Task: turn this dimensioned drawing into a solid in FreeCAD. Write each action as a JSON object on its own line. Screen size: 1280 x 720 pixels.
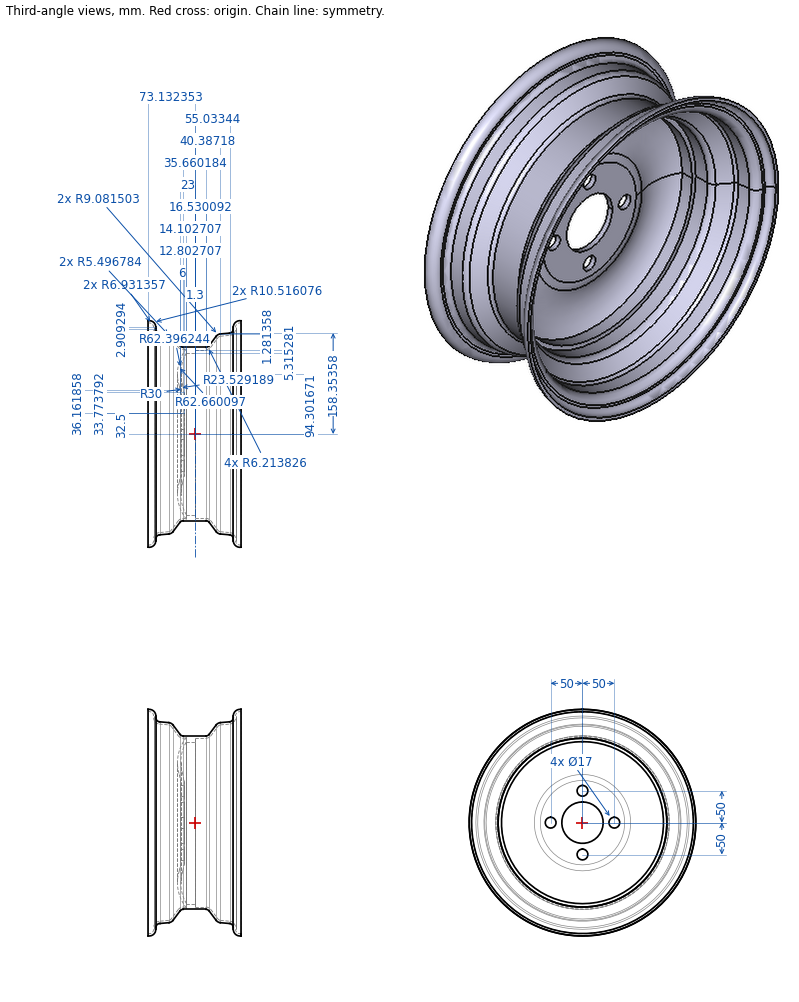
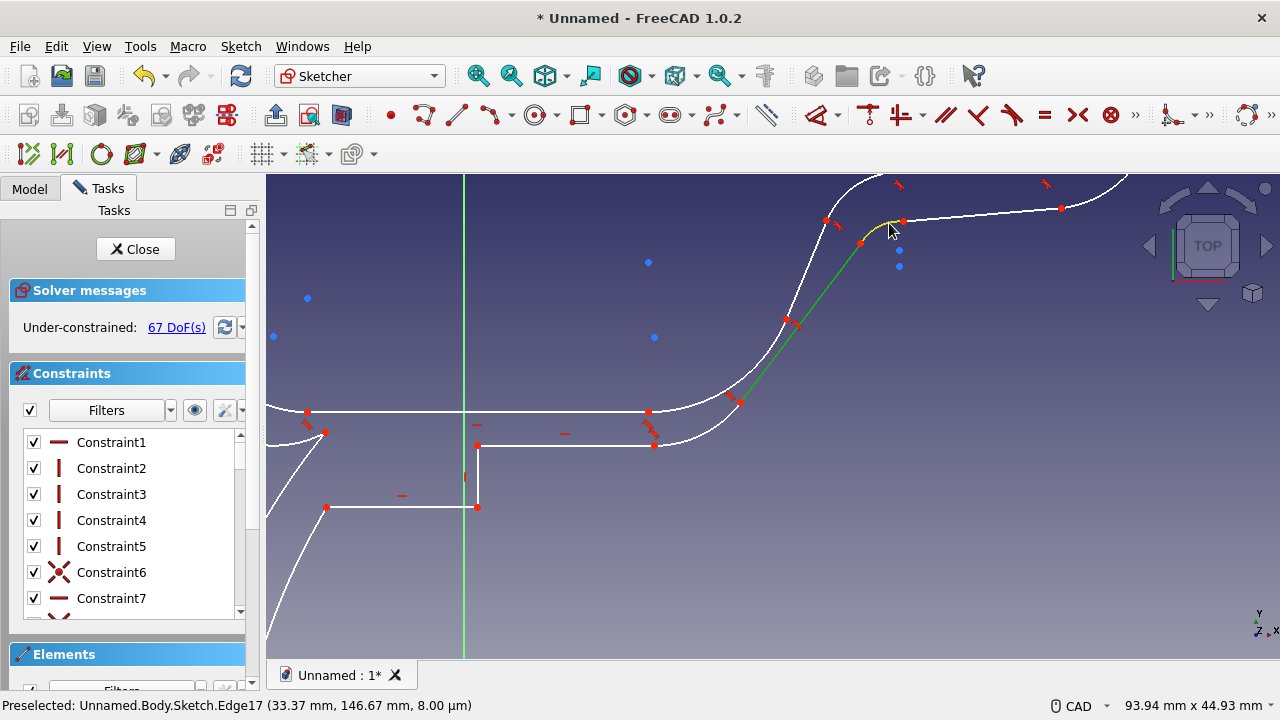
{"action": "left_click", "coordinate": [888, 223]}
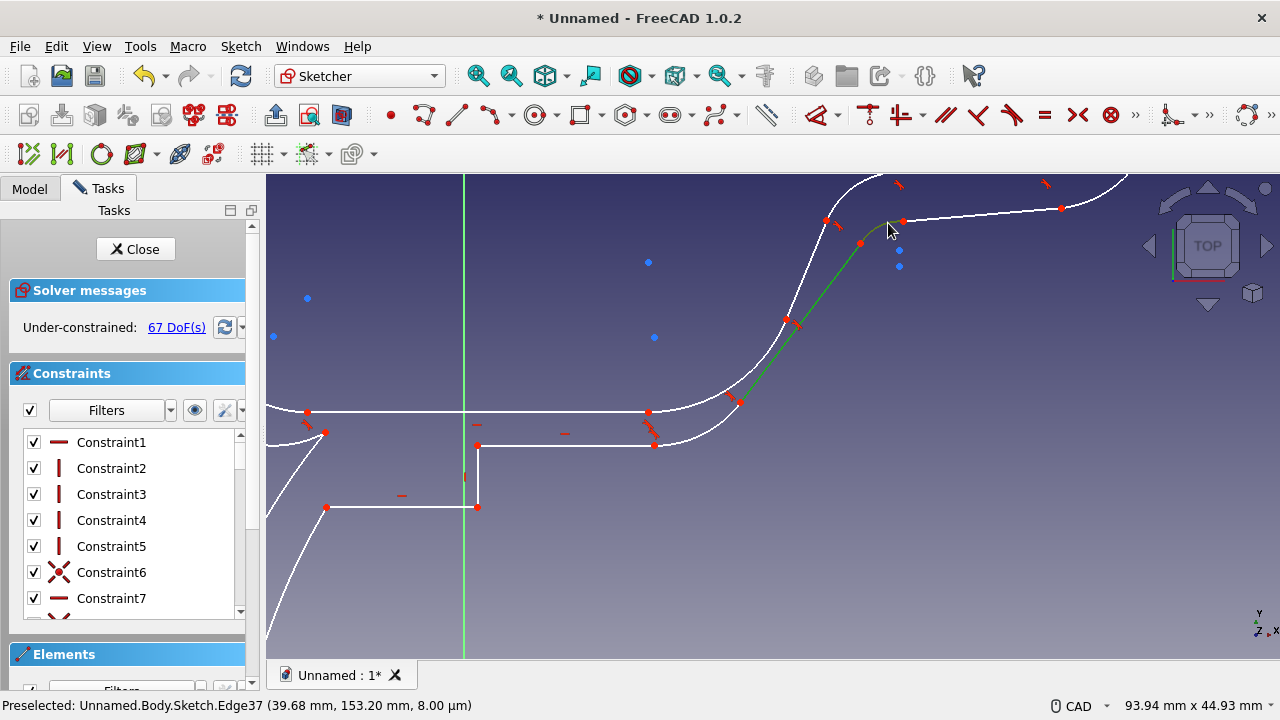
{"action": "key", "text": "t"}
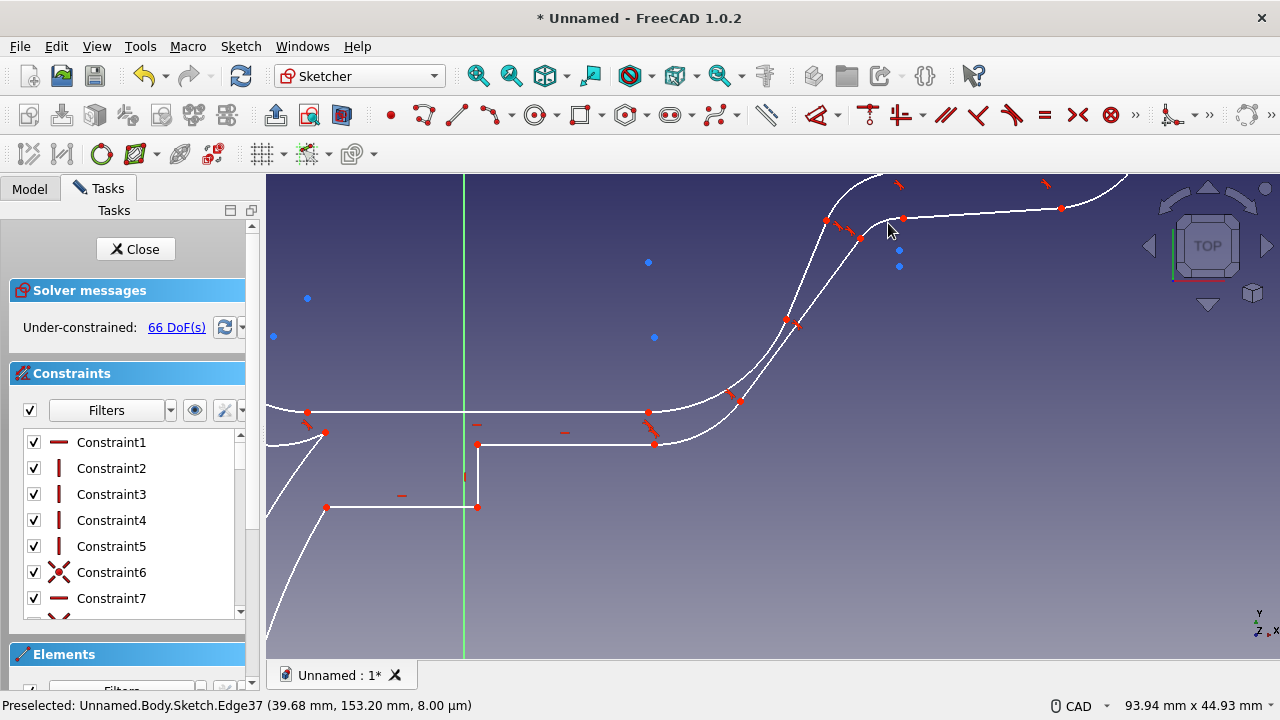
{"action": "scroll", "coordinate": [752, 318], "scroll_direction": "down", "scroll_amount": 9}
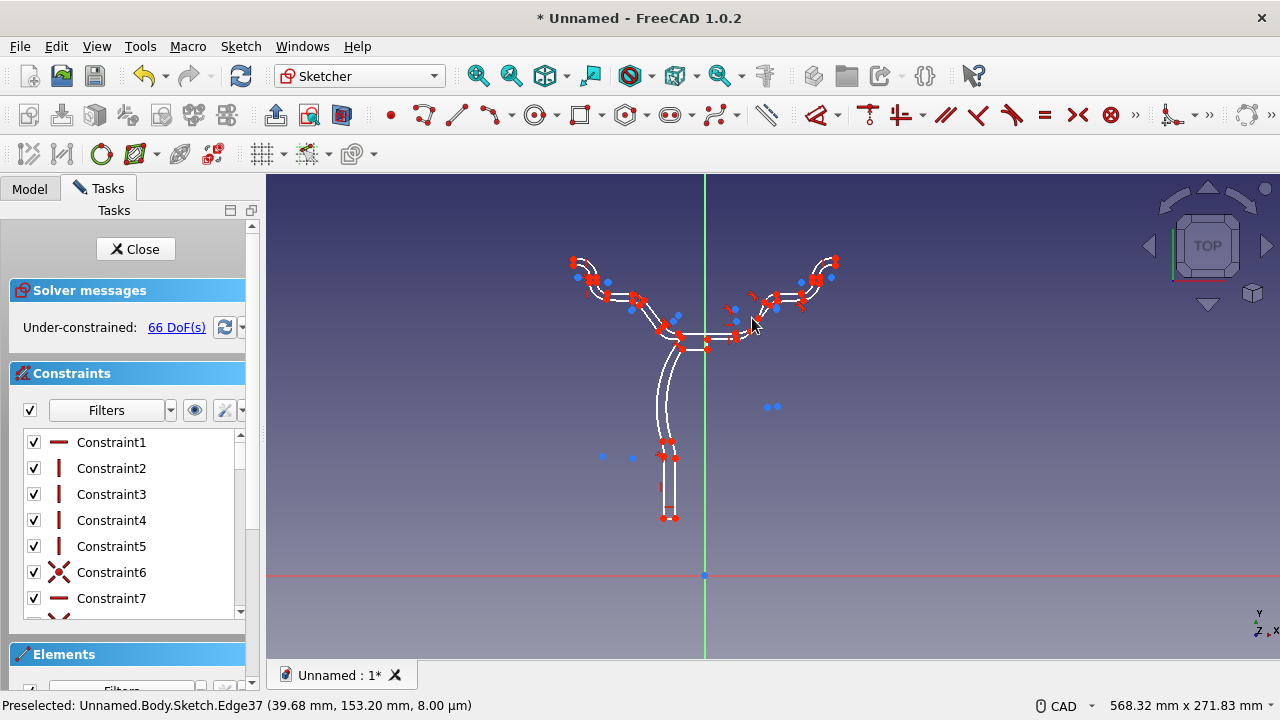
{"action": "scroll", "coordinate": [785, 301], "scroll_direction": "up", "scroll_amount": 4}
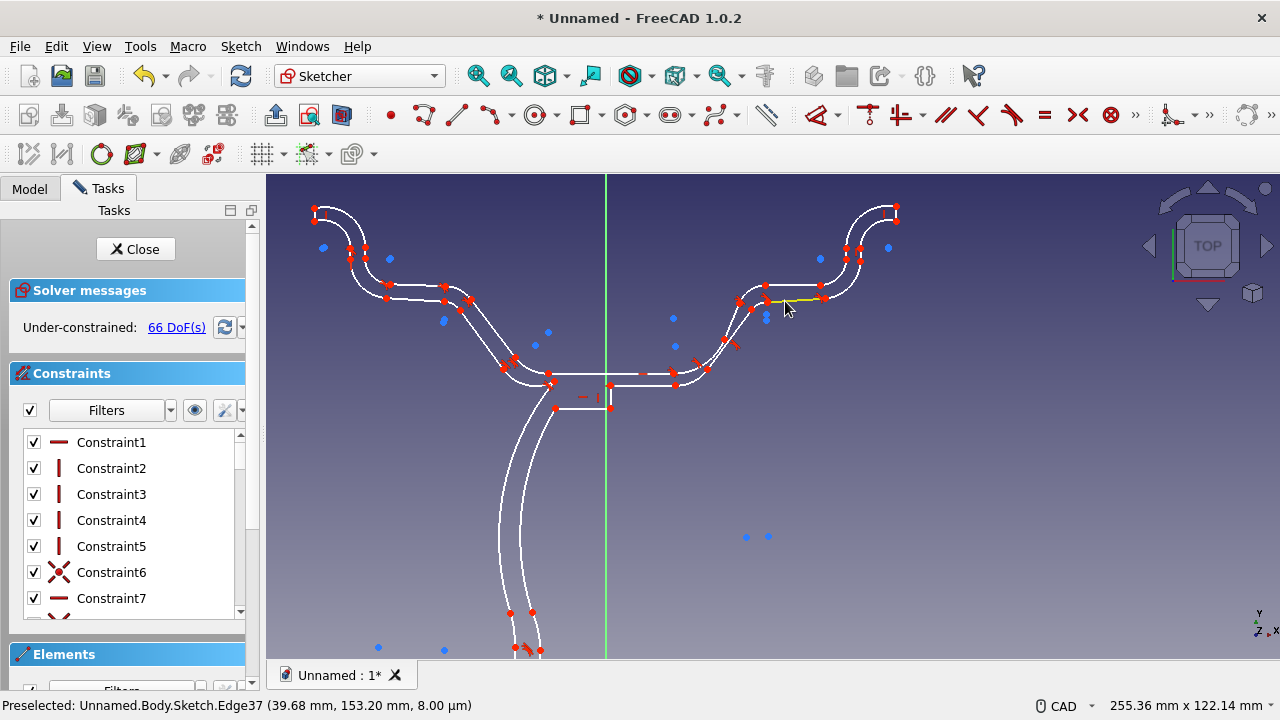
{"action": "left_click", "coordinate": [785, 301]}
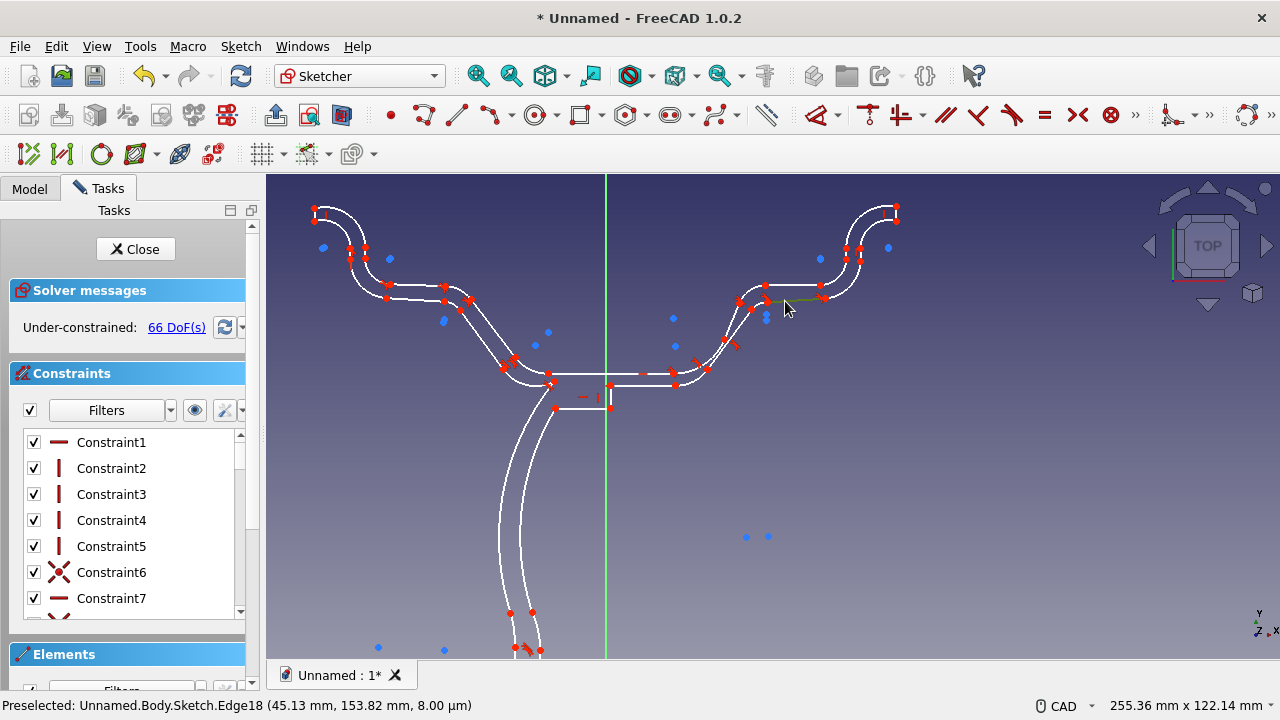
{"action": "scroll", "coordinate": [759, 304], "scroll_direction": "up", "scroll_amount": 3}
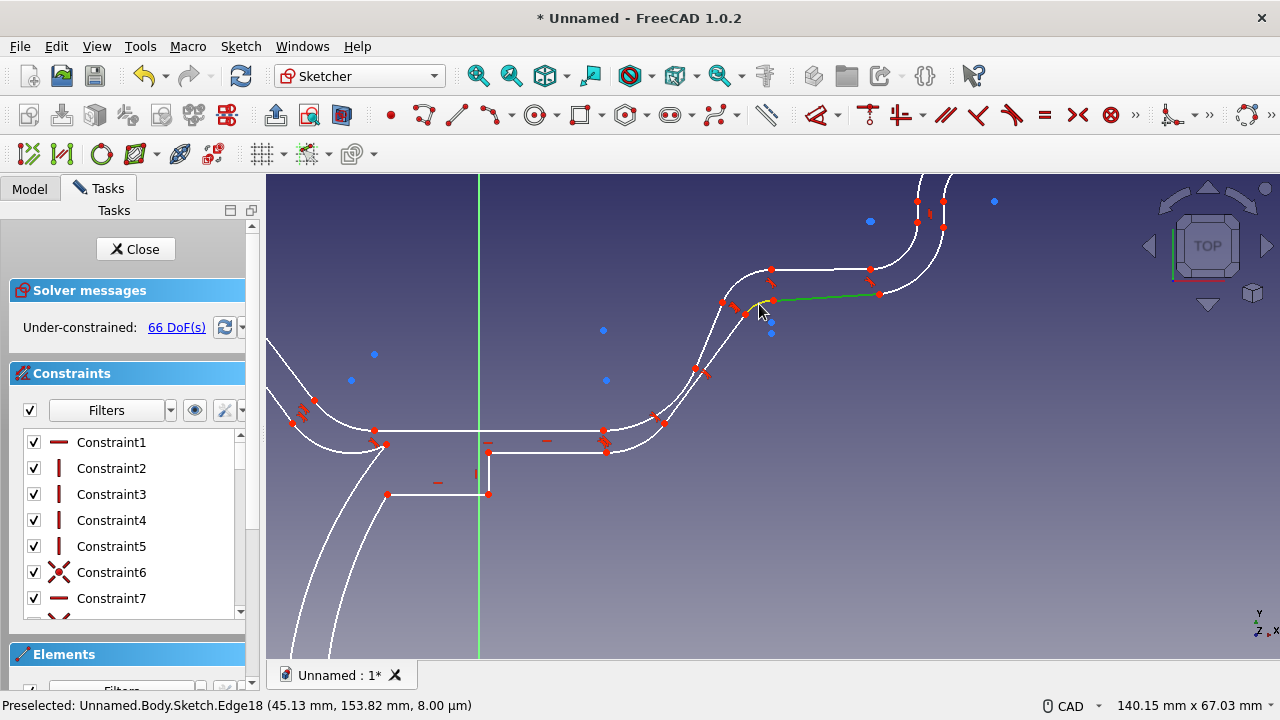
{"action": "left_click", "coordinate": [758, 304]}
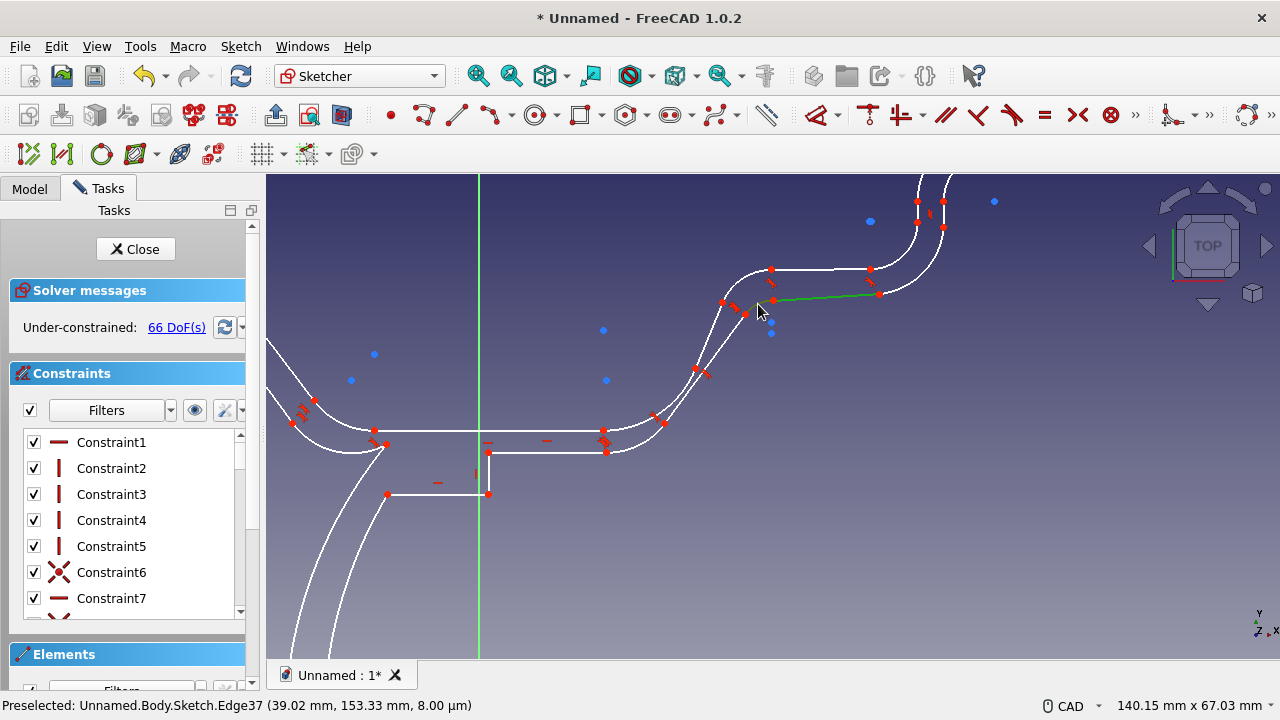
{"action": "key", "text": "t"}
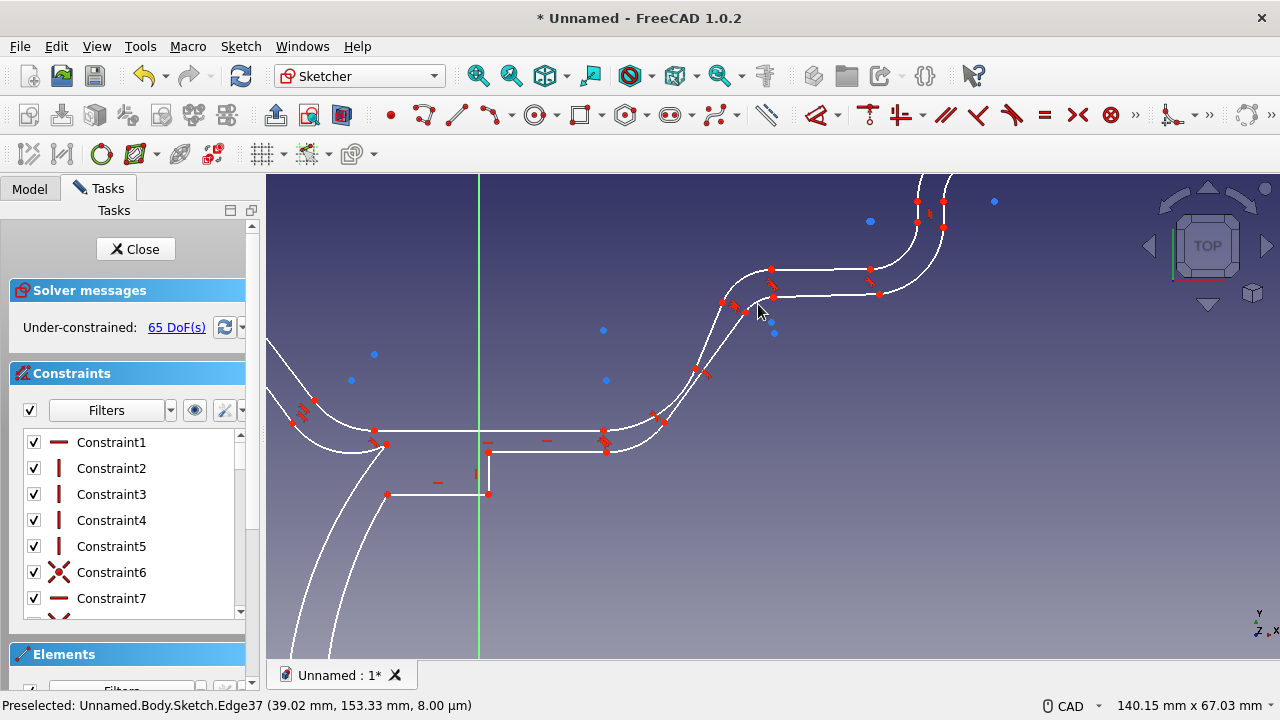
{"action": "left_click", "coordinate": [806, 296]}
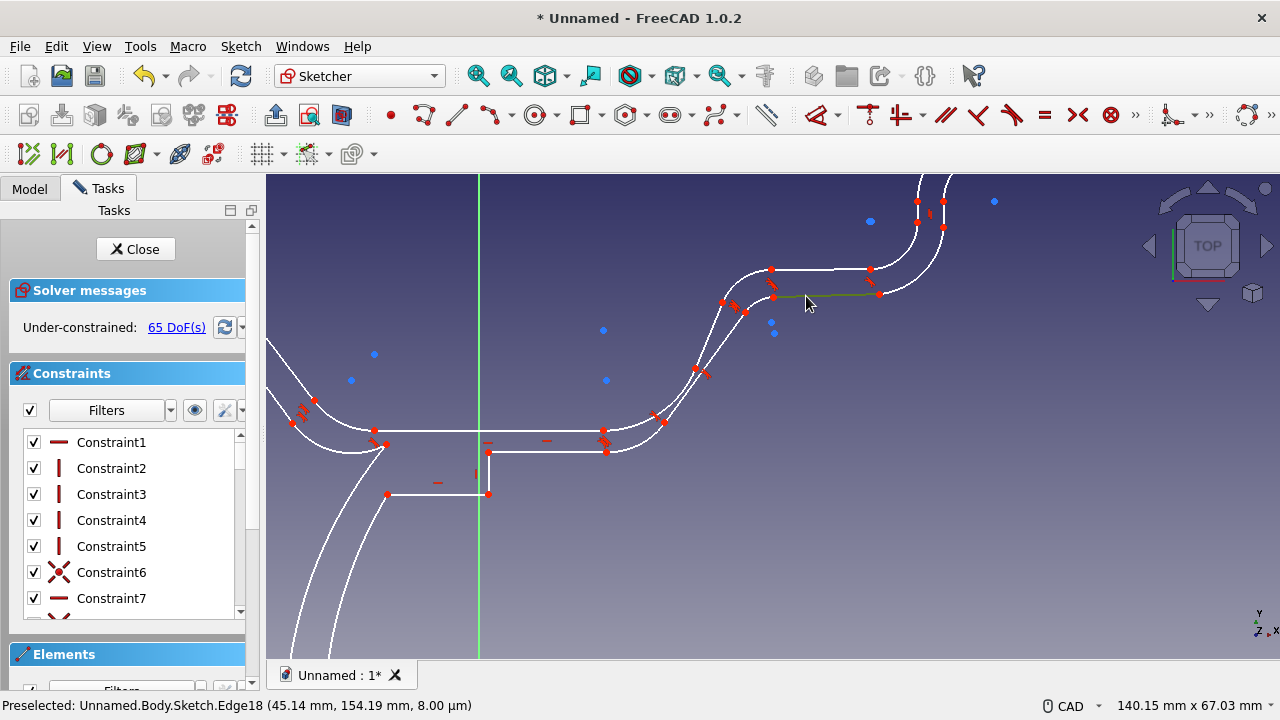
{"action": "left_click", "coordinate": [908, 285]}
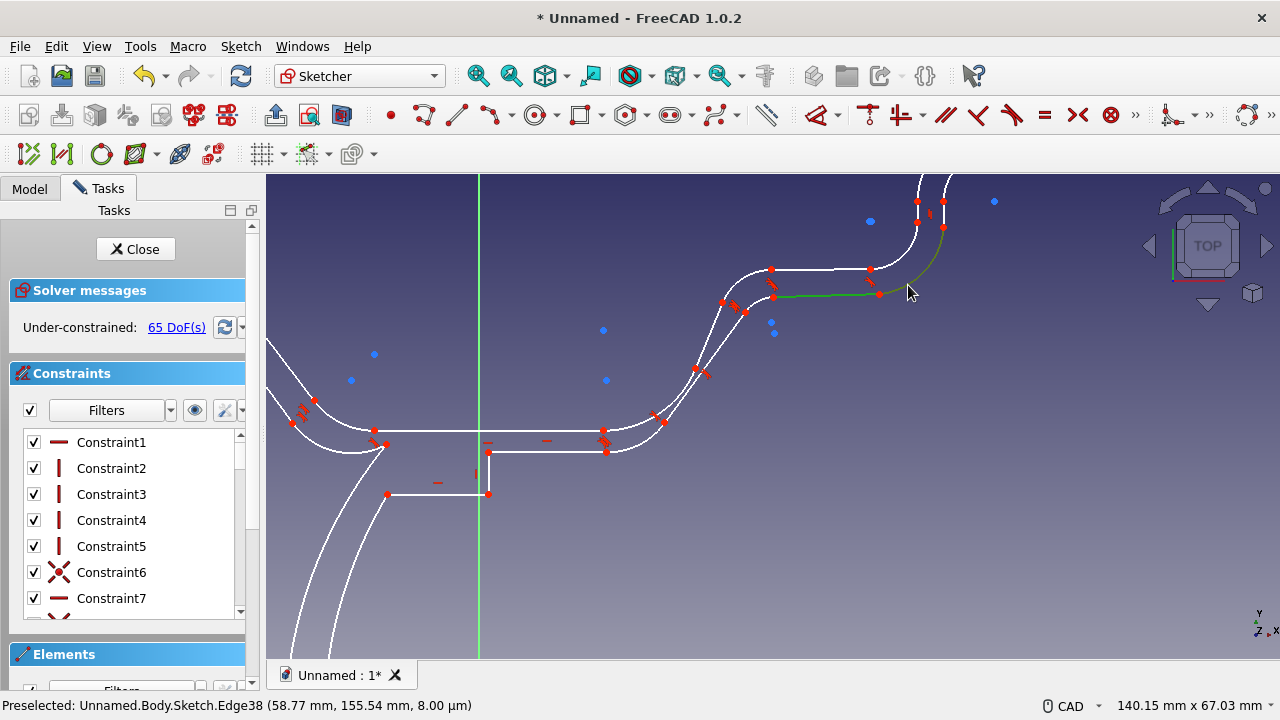
{"action": "key", "text": "t"}